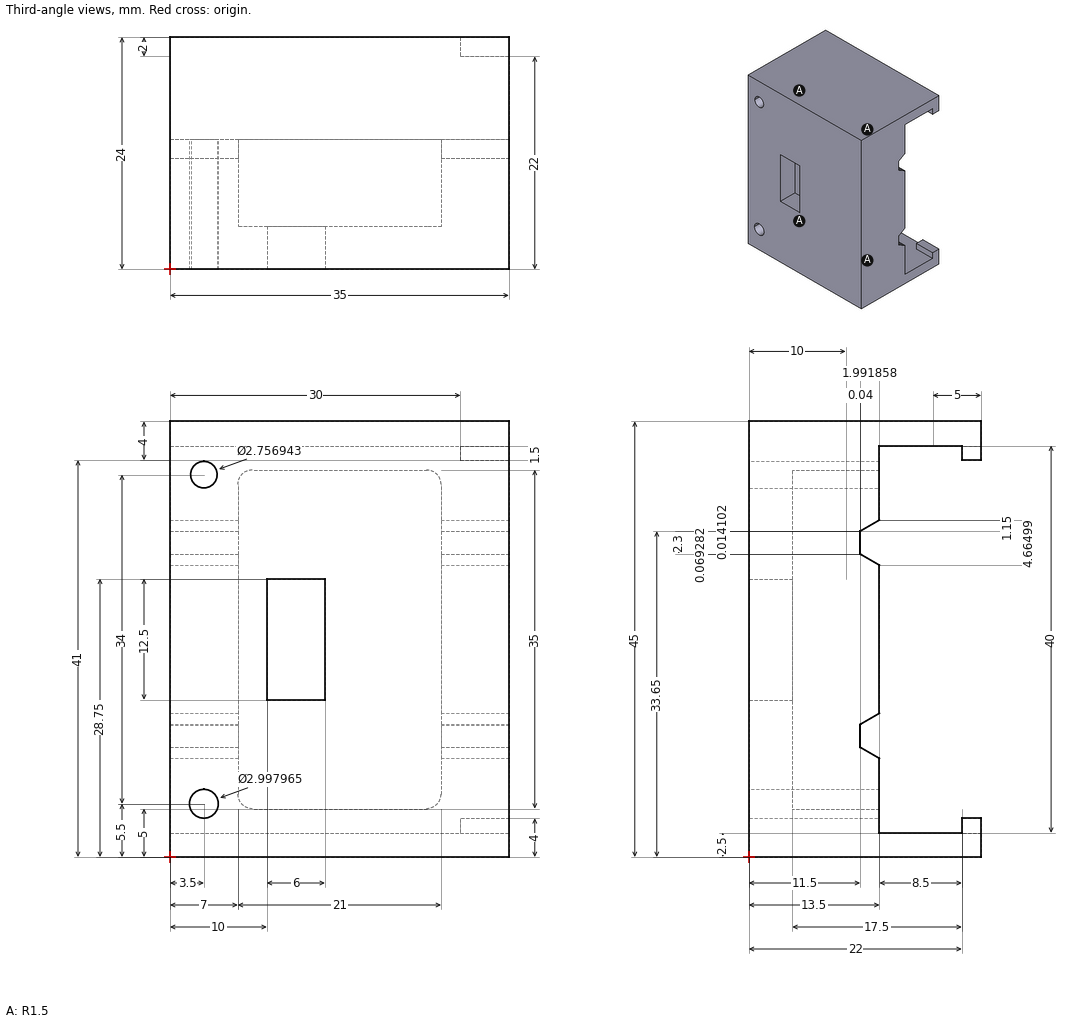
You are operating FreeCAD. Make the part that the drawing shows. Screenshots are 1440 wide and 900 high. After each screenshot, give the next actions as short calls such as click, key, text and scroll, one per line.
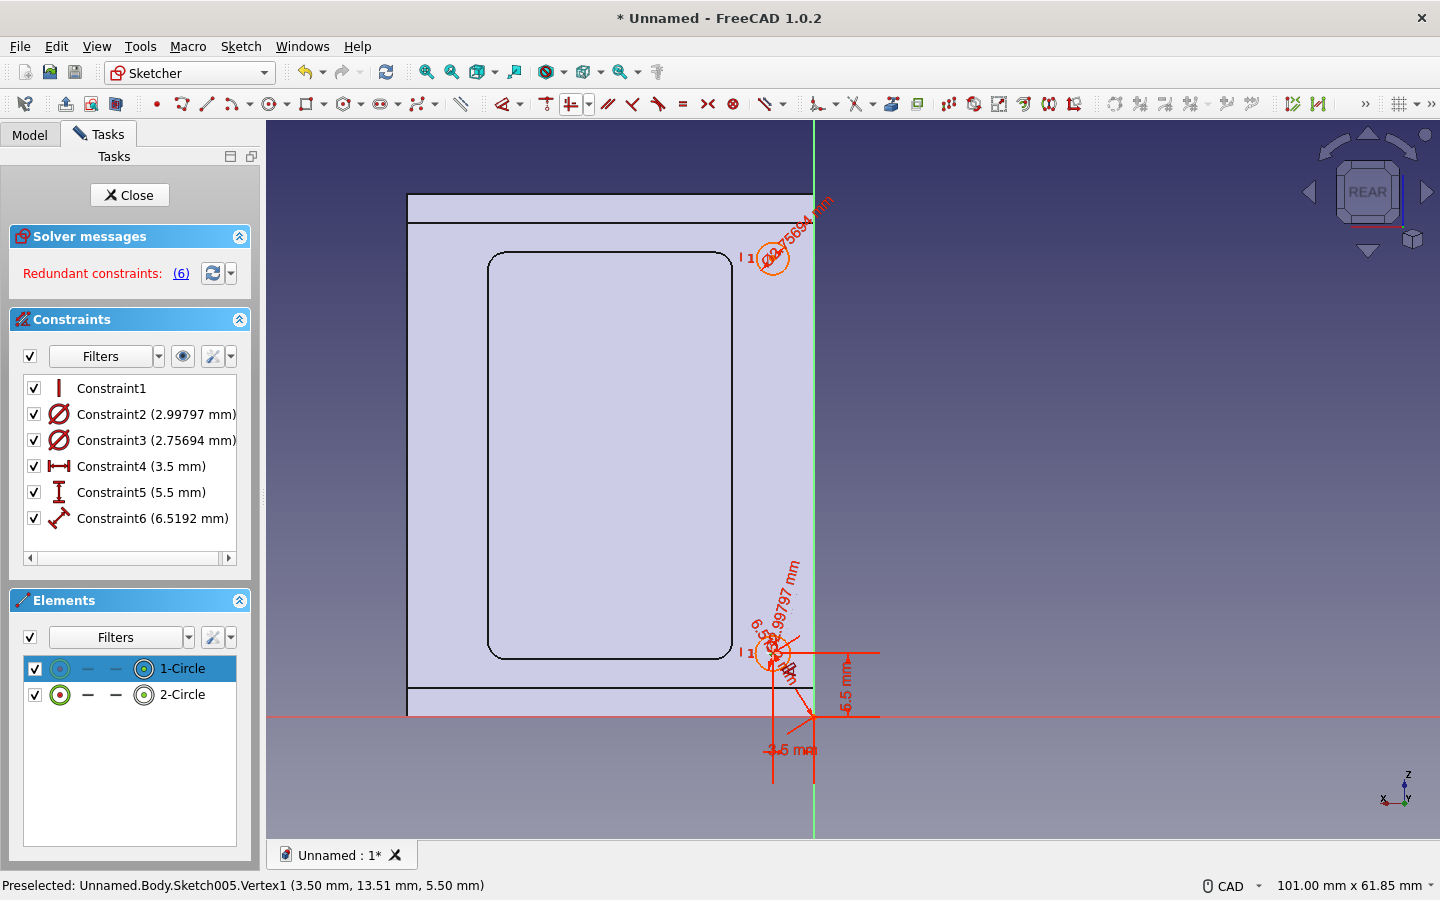
click(773, 259)
click(739, 456)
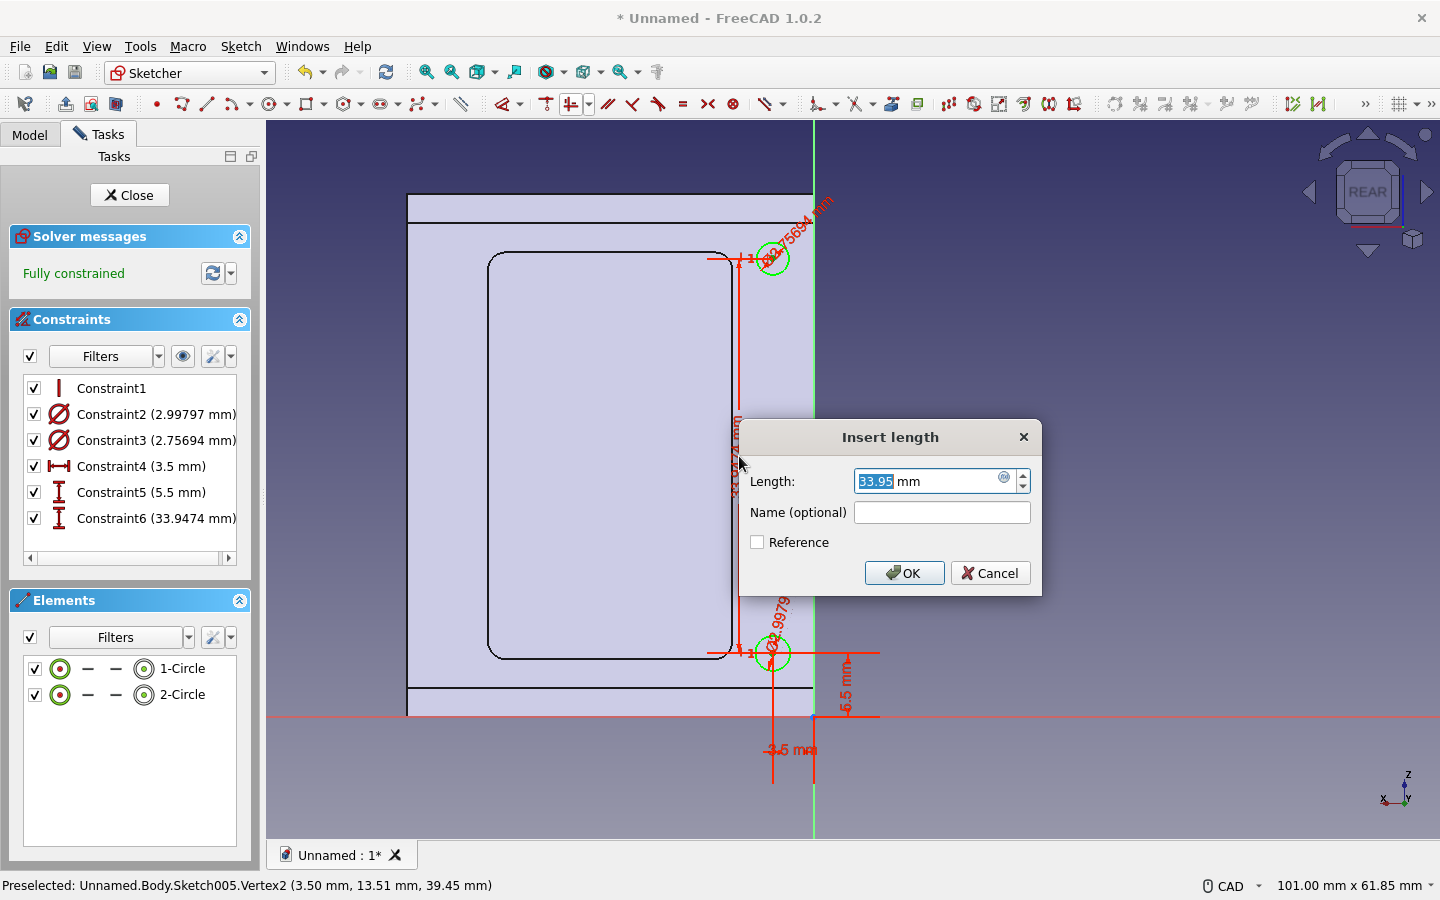
text(34)
key(Return)
key(Escape)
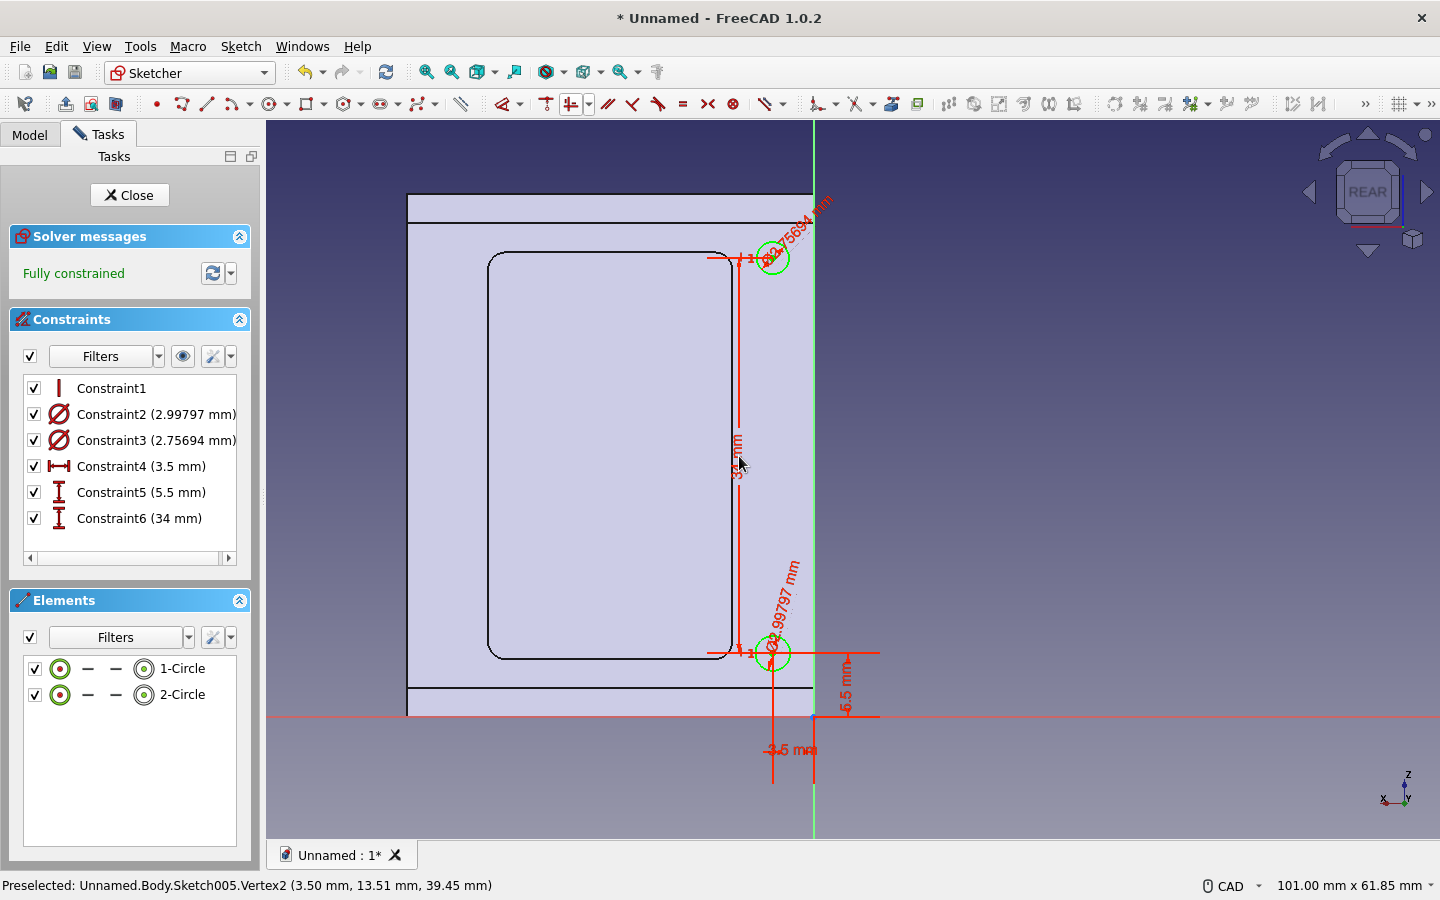
click(130, 195)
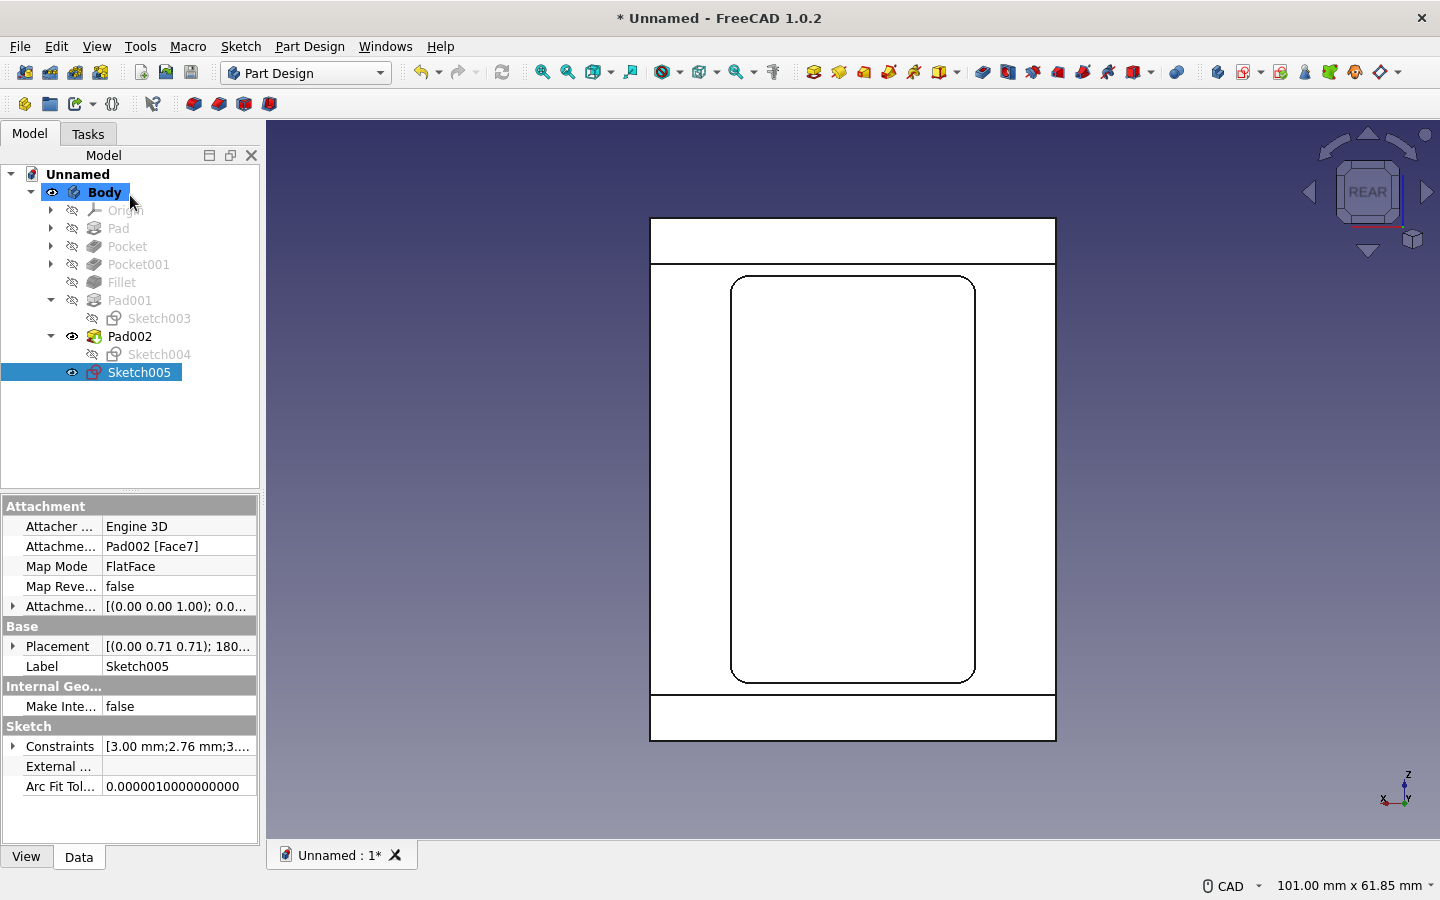
click(983, 72)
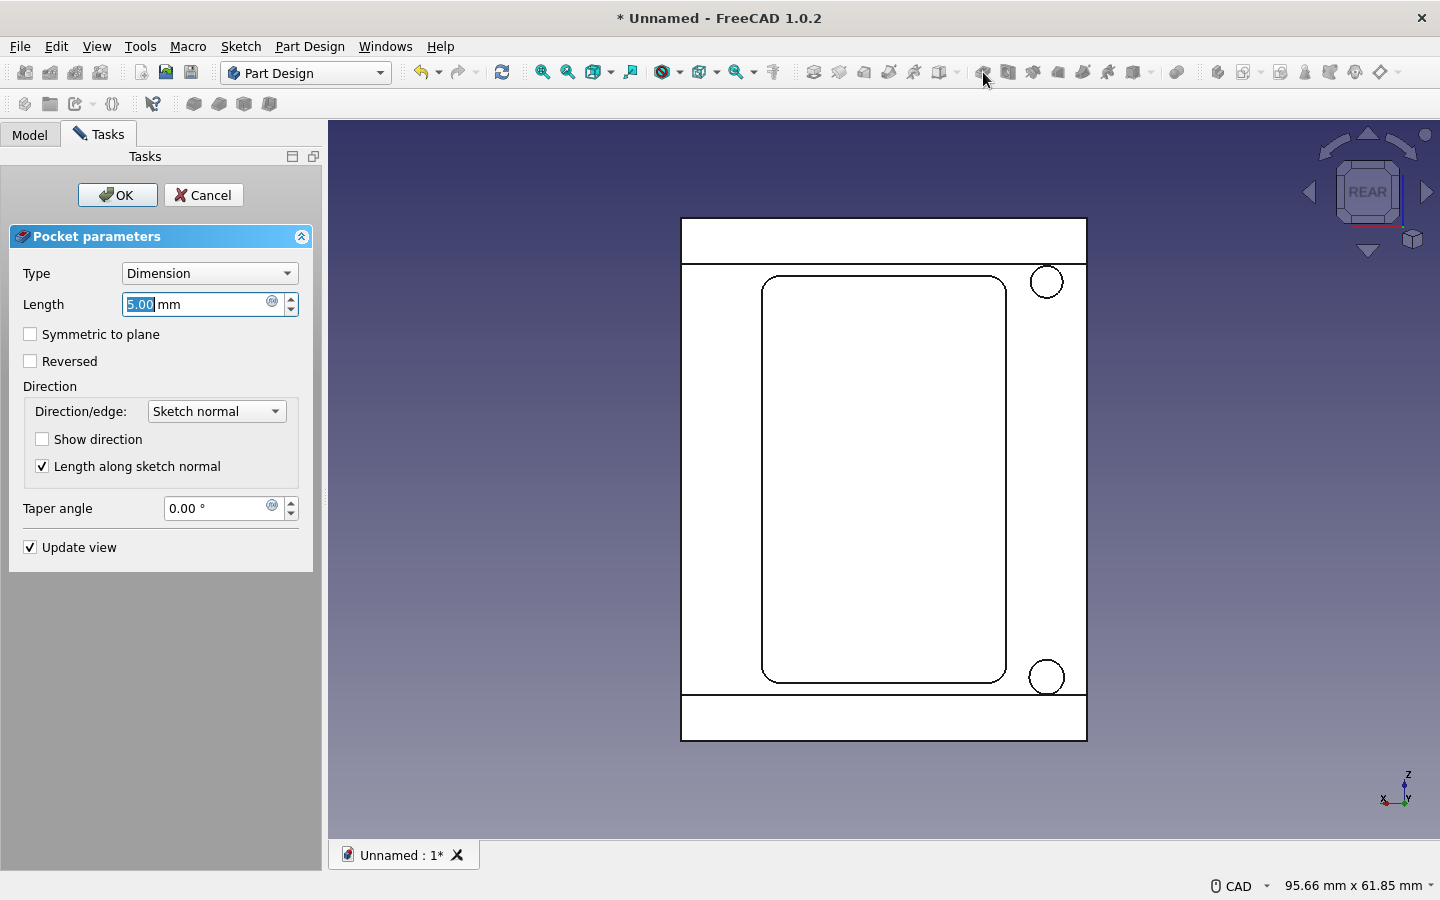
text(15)
key(Tab)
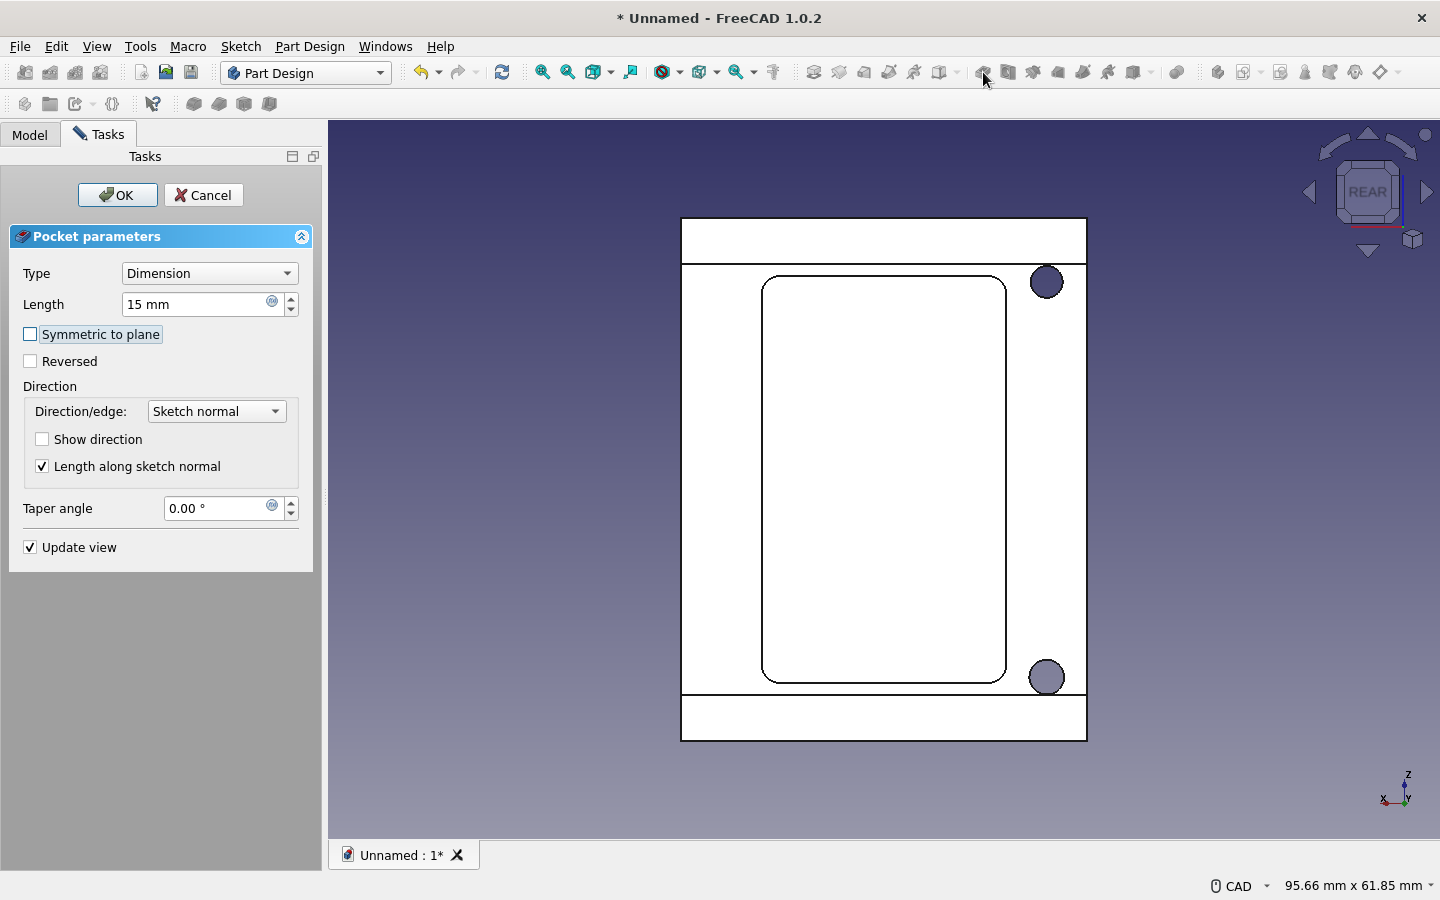
click(118, 195)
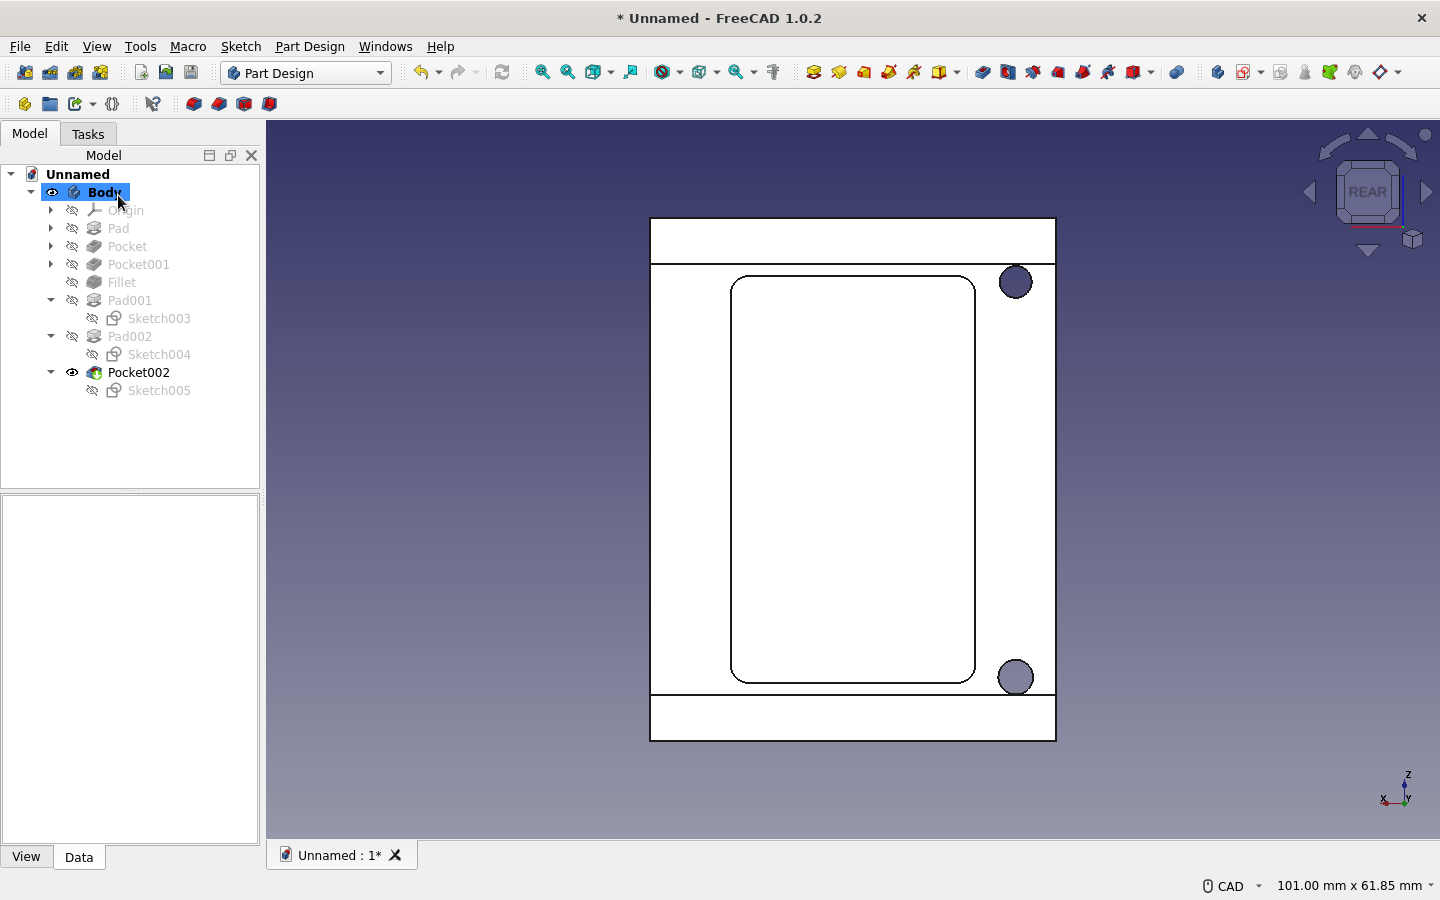
click(679, 240)